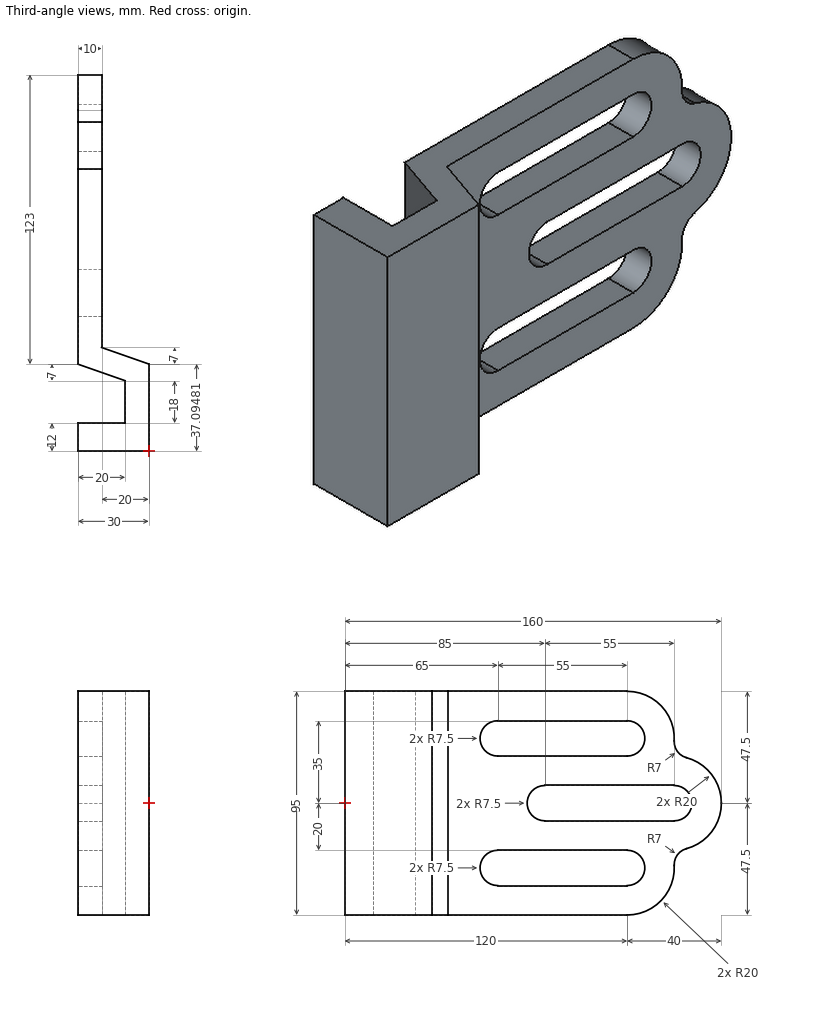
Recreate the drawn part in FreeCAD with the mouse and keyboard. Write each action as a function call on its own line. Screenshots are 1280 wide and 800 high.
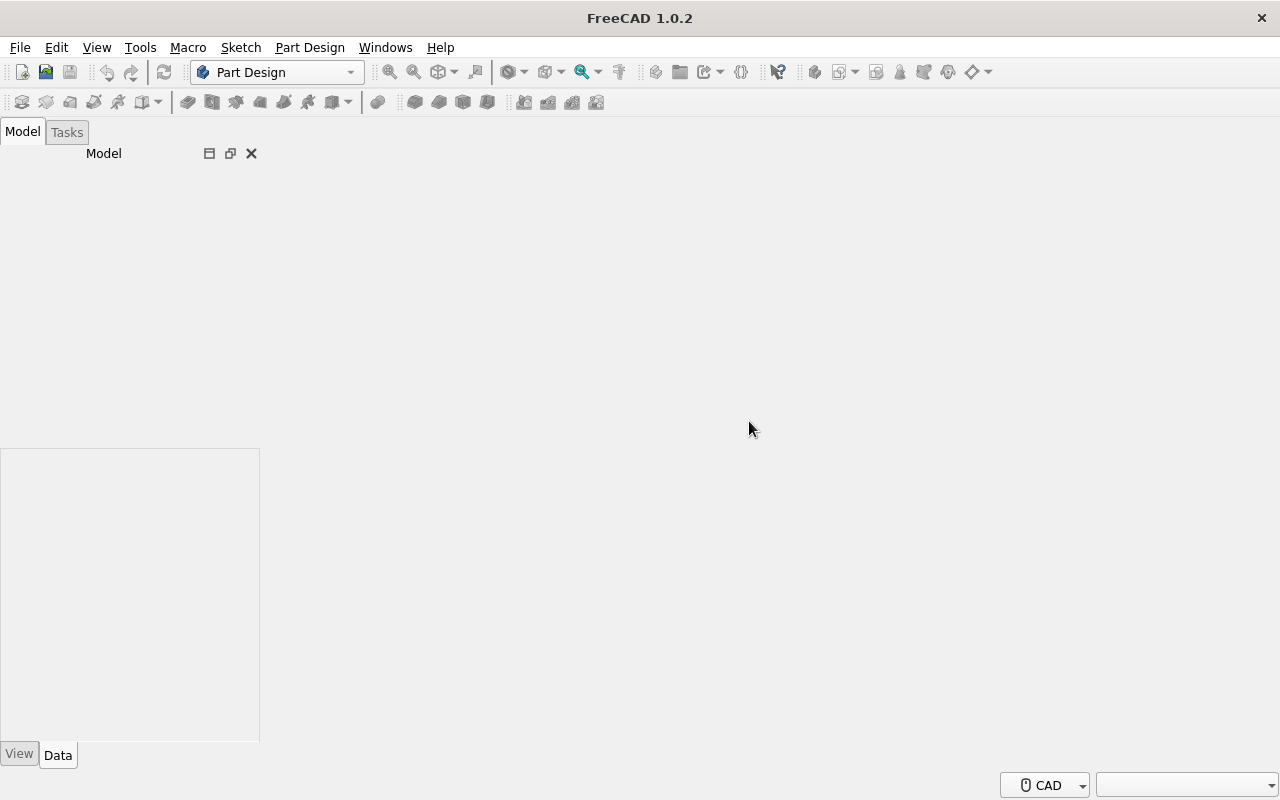
click(22, 72)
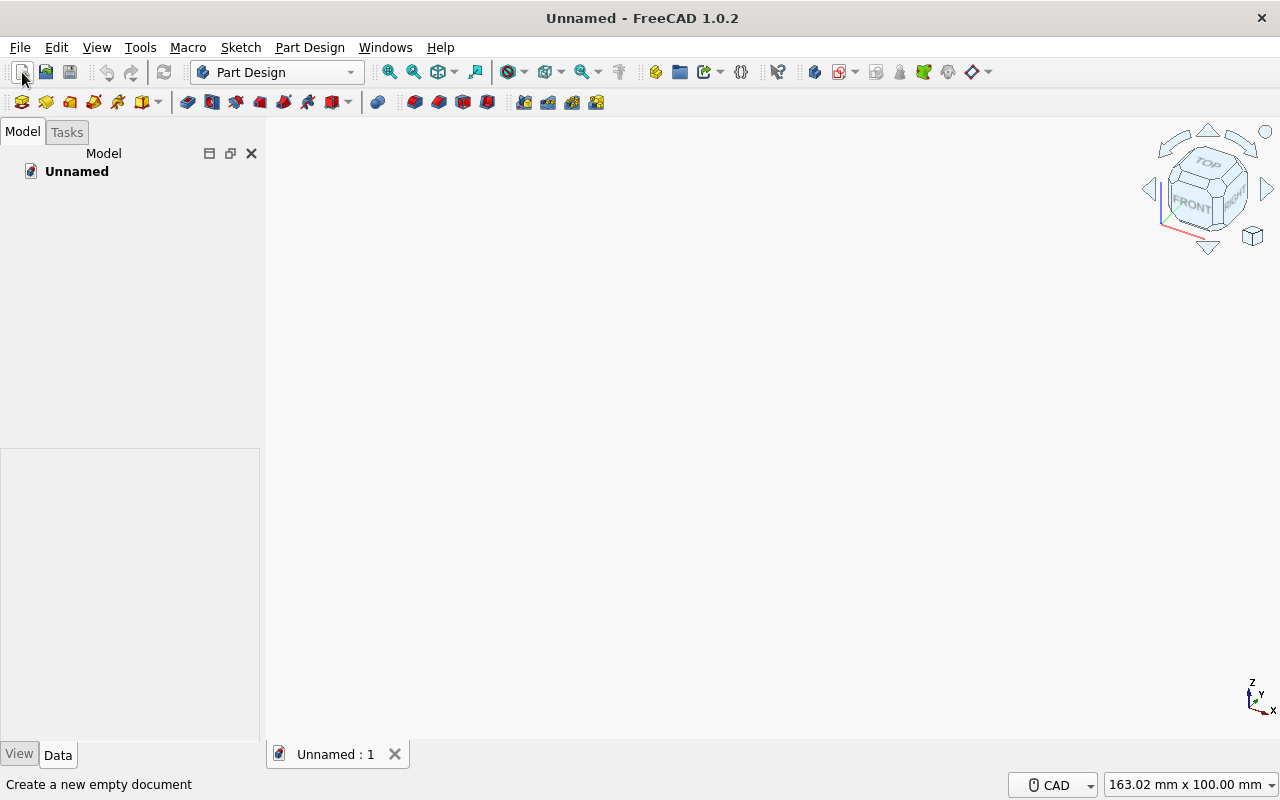
click(840, 72)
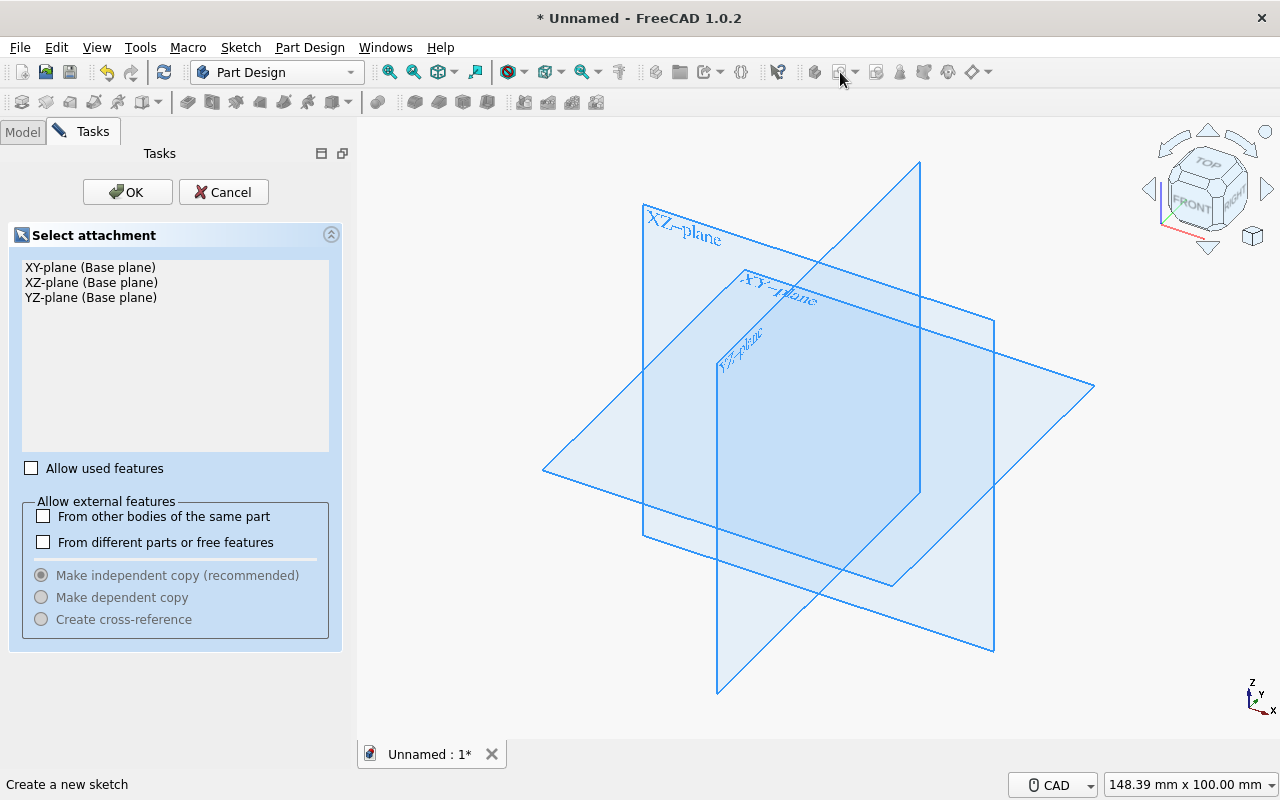
click(82, 268)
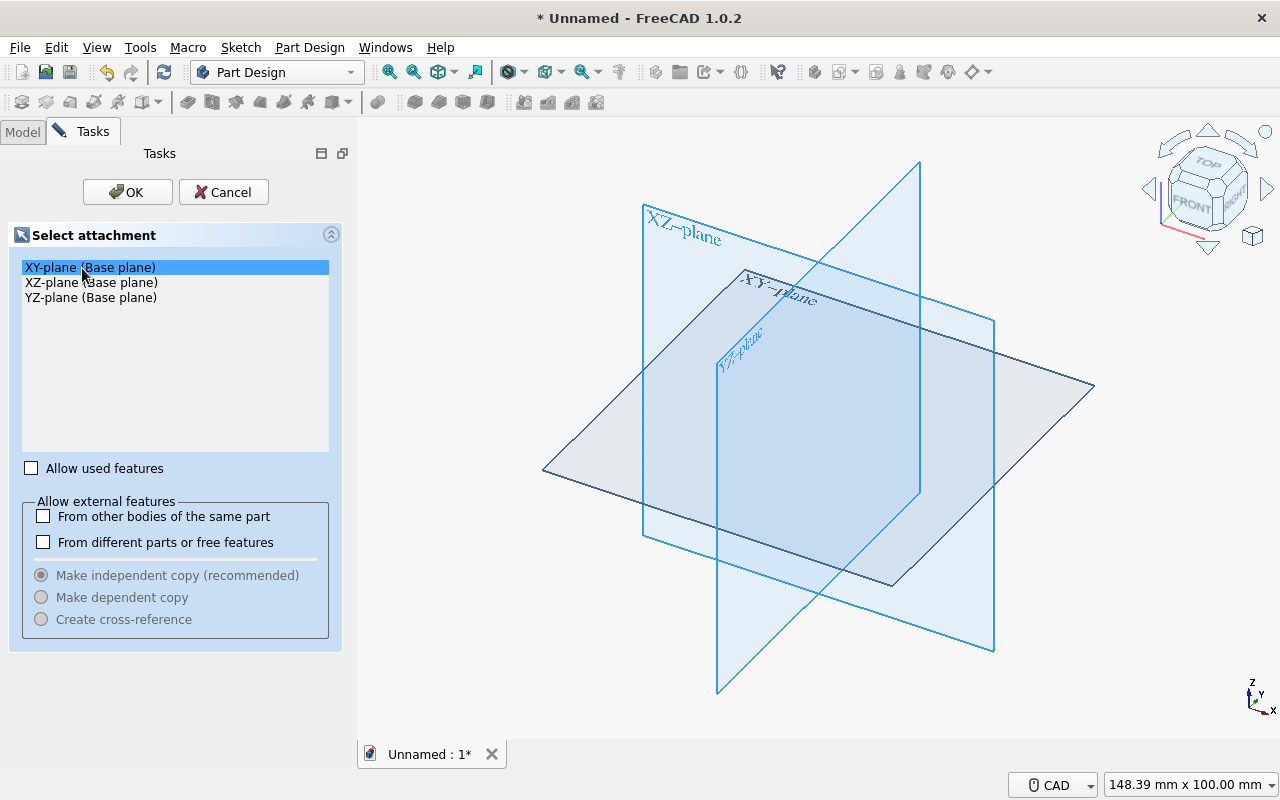
click(128, 192)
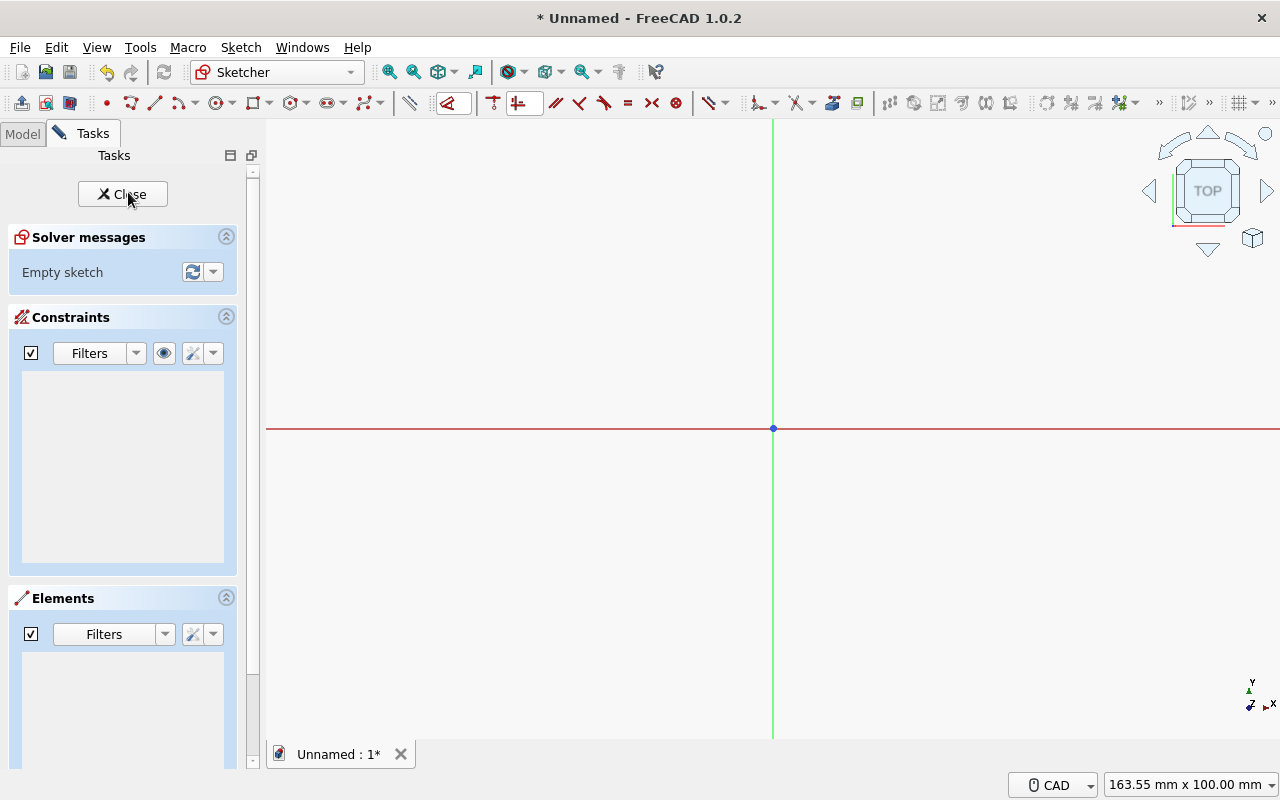
scroll(719, 711, down, 5)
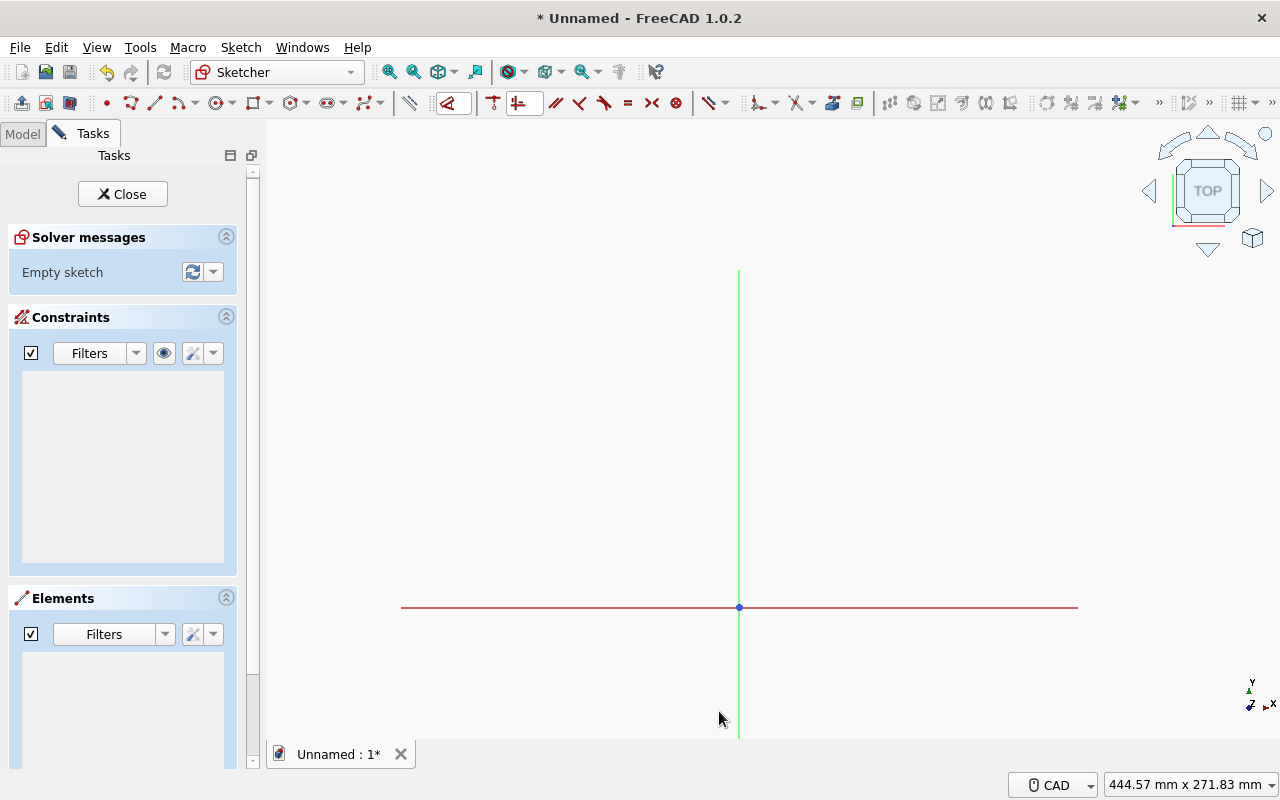
click(132, 104)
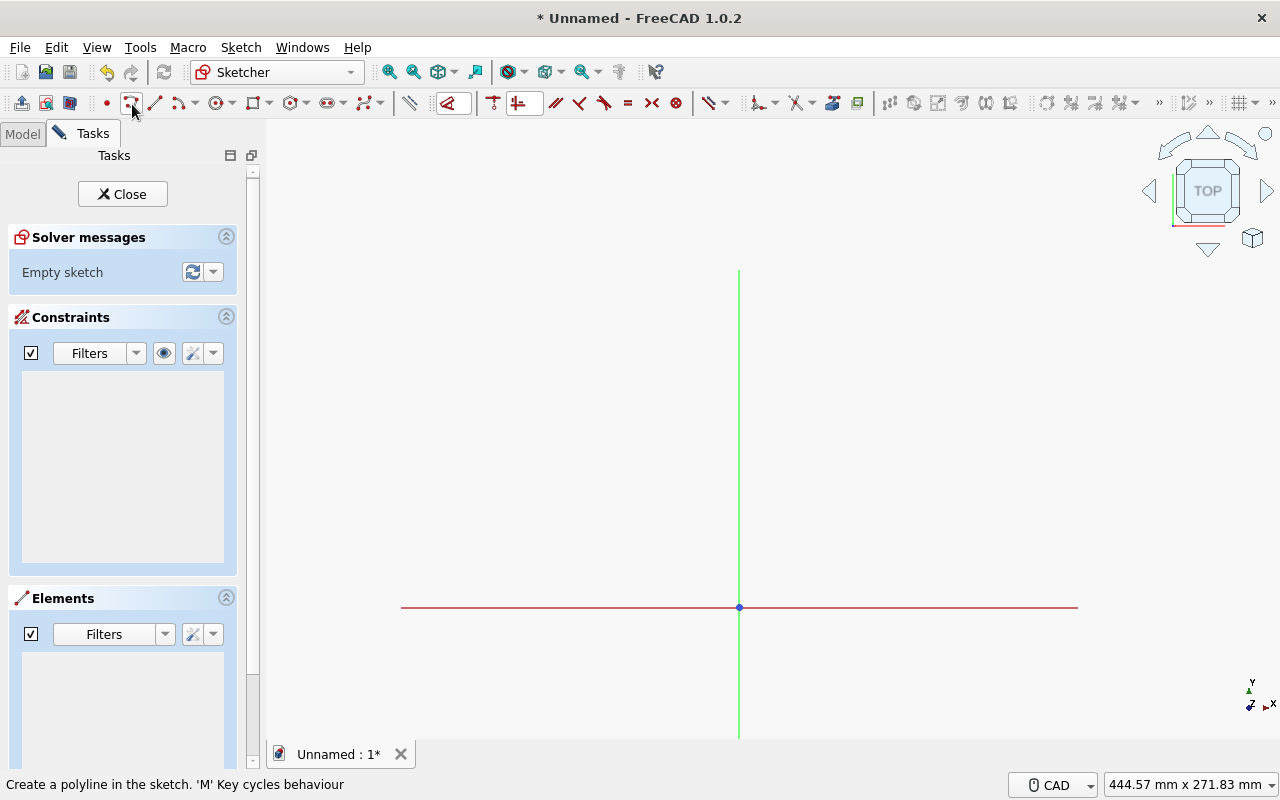
click(739, 608)
click(730, 523)
click(694, 507)
click(694, 243)
click(671, 243)
click(671, 523)
click(716, 539)
click(716, 580)
click(671, 580)
click(671, 599)
click(739, 608)
key(Escape)
key(Escape)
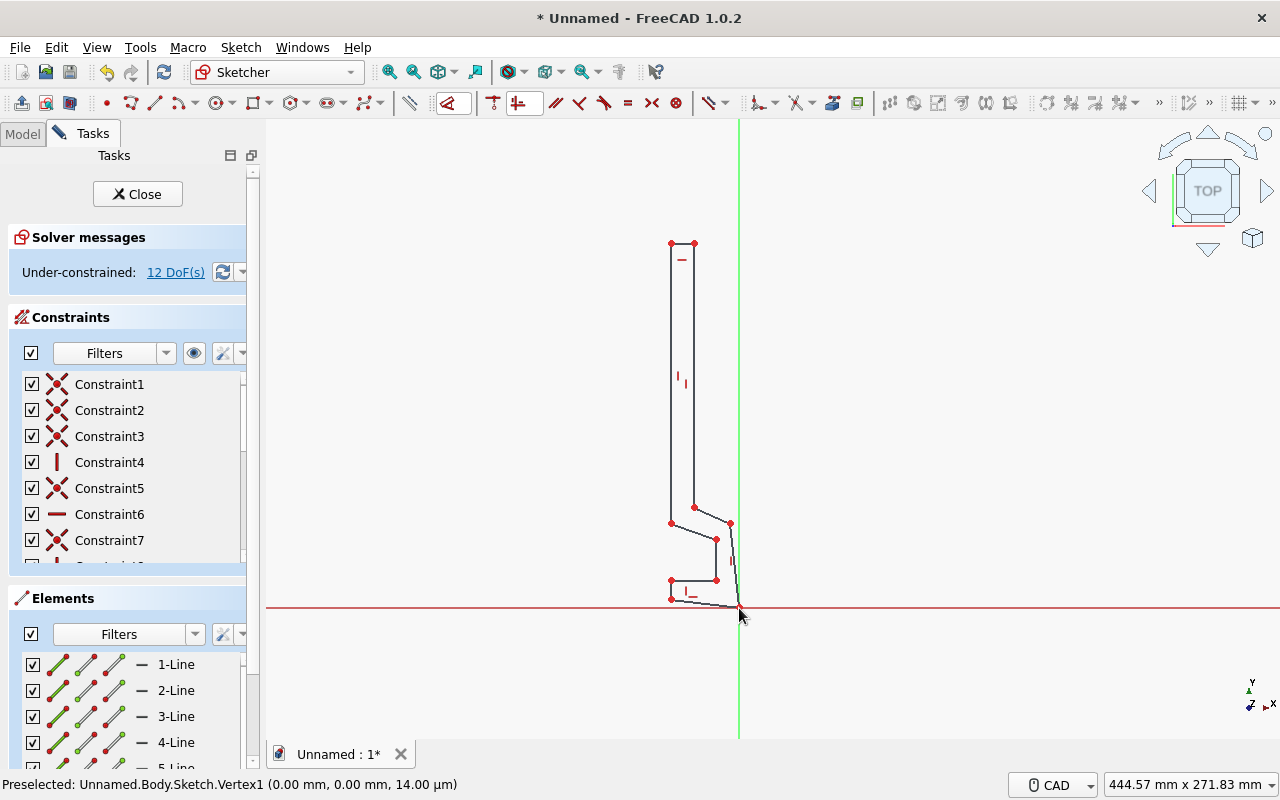
click(736, 583)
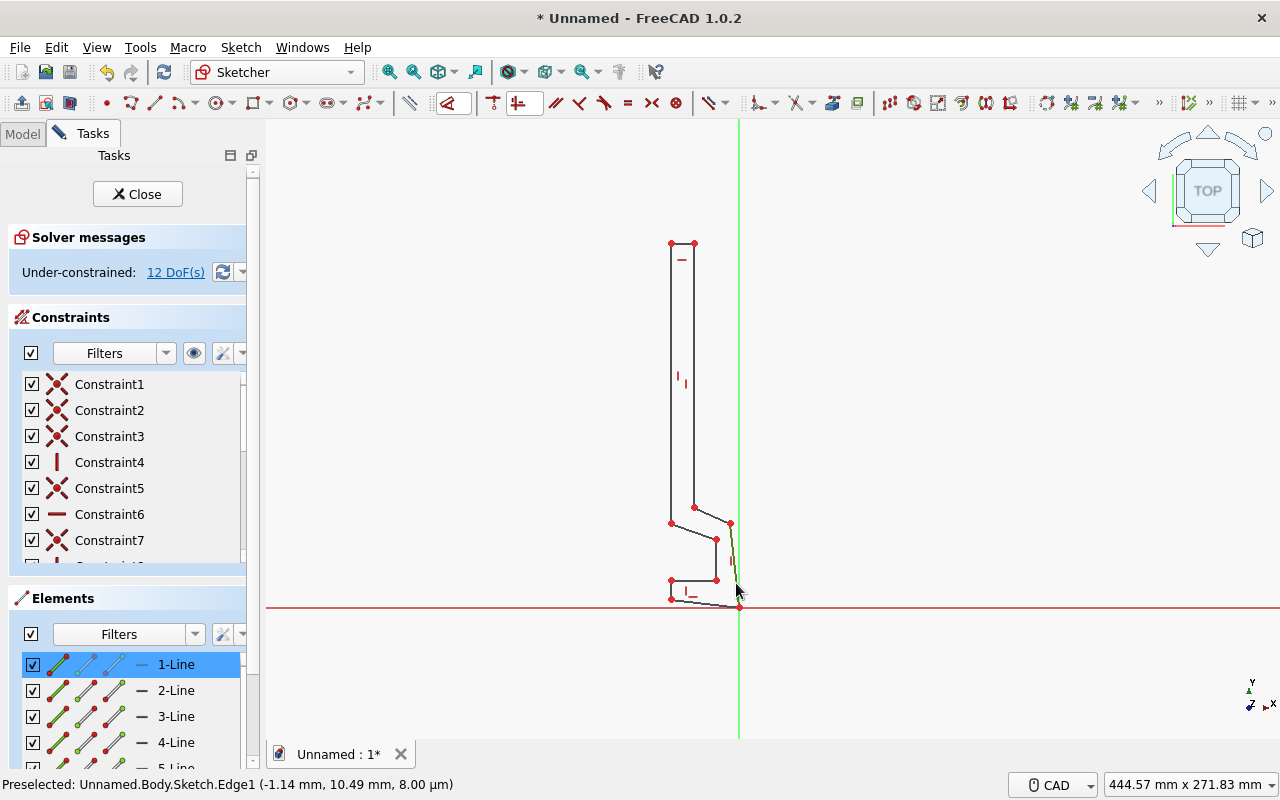
click(538, 104)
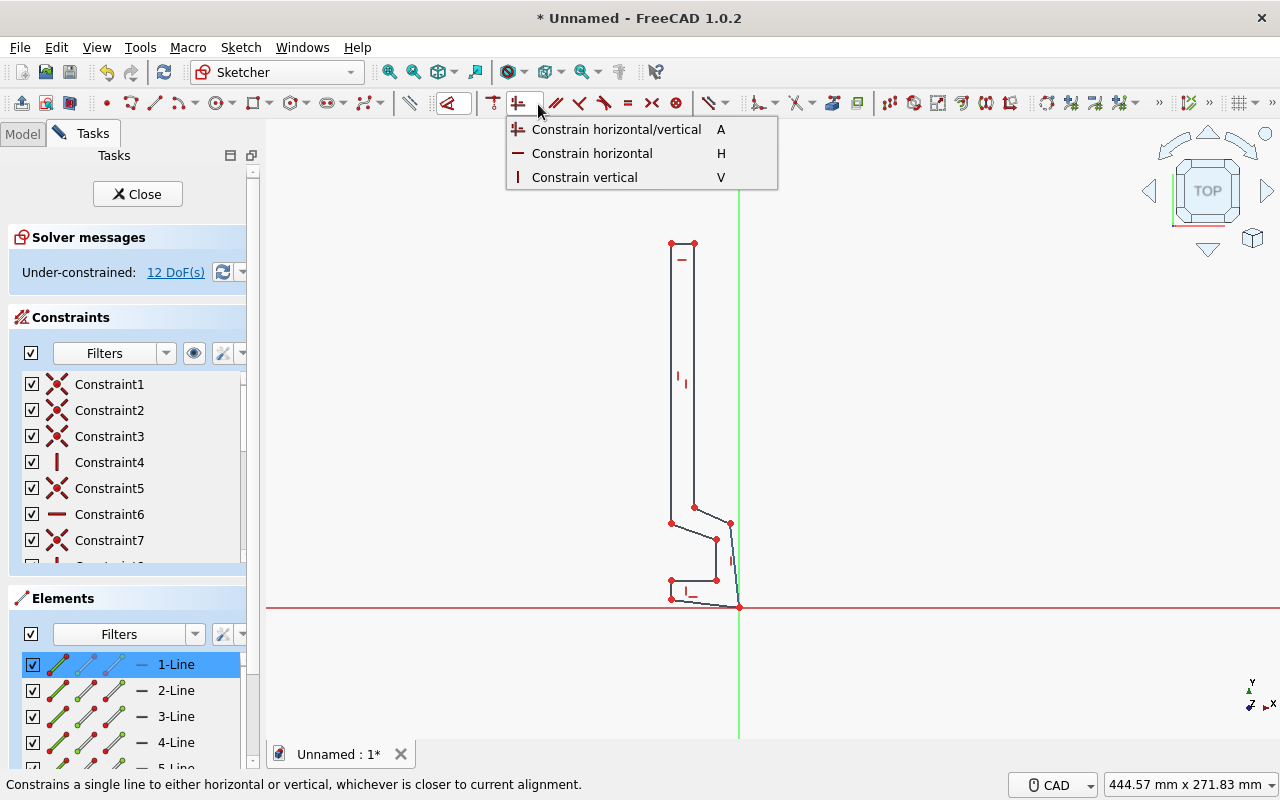
click(642, 177)